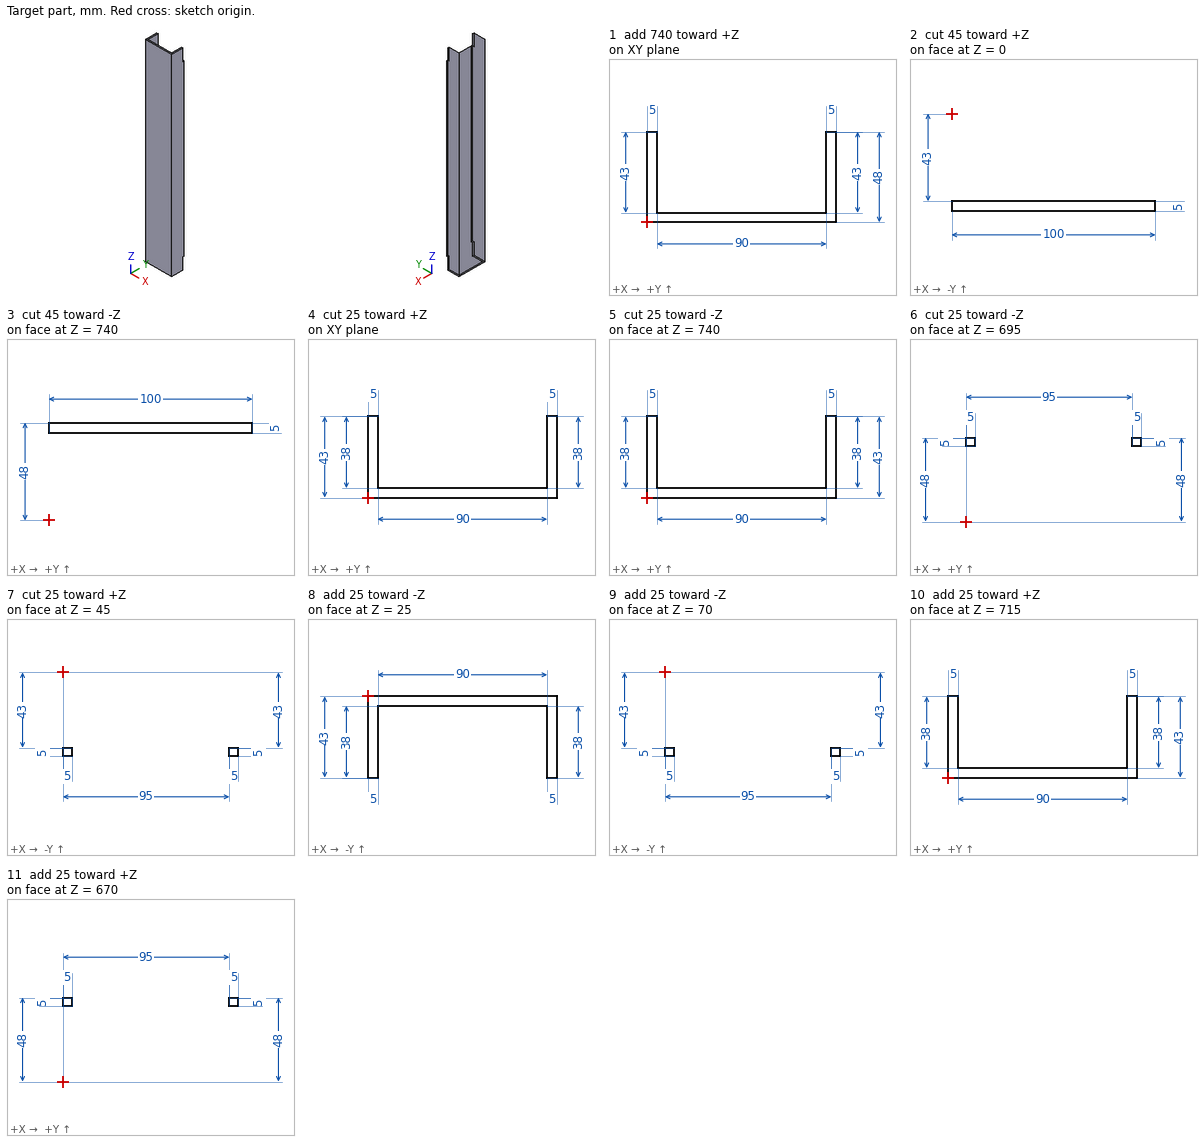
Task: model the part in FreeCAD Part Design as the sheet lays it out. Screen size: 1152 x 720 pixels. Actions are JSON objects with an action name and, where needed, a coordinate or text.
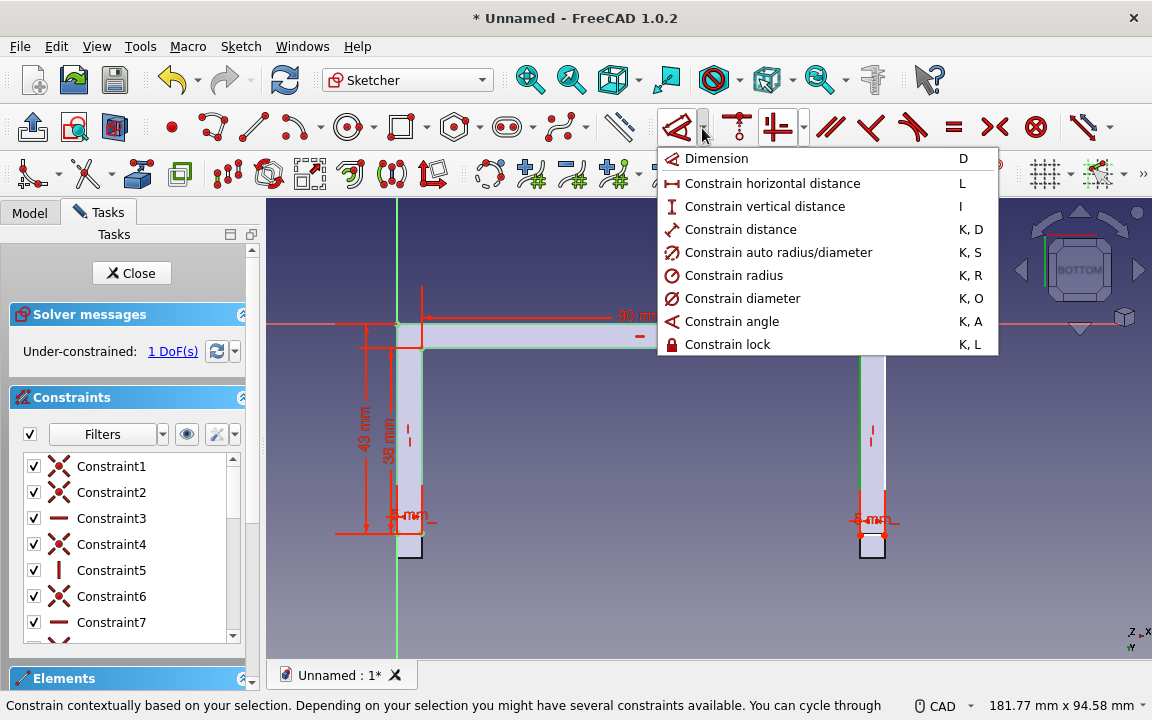
{"action": "left_click", "coordinate": [828, 206]}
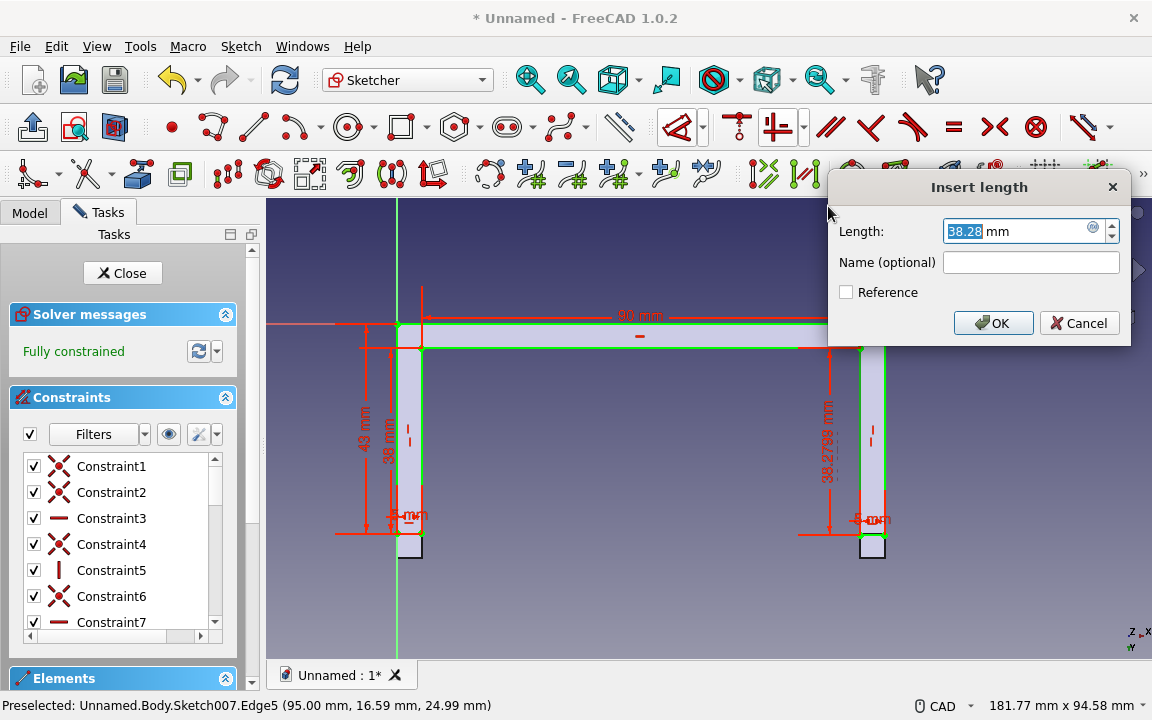
{"action": "type", "text": "38"}
{"action": "key", "text": "Return"}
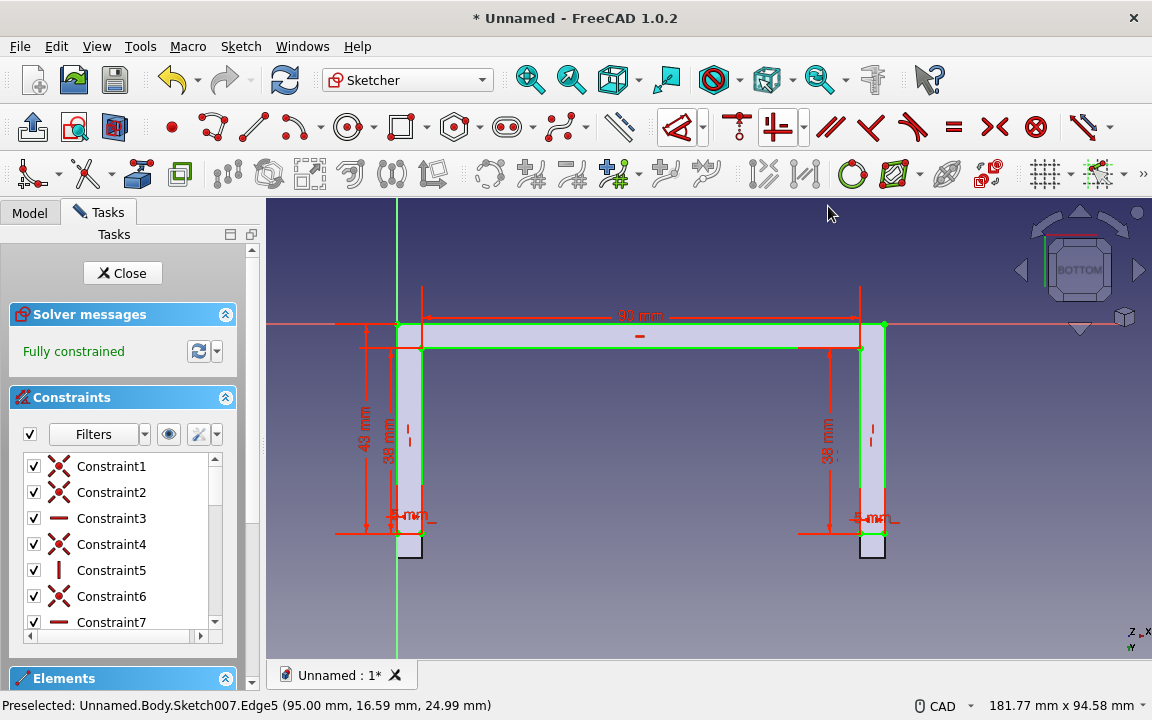
{"action": "left_click", "coordinate": [123, 273]}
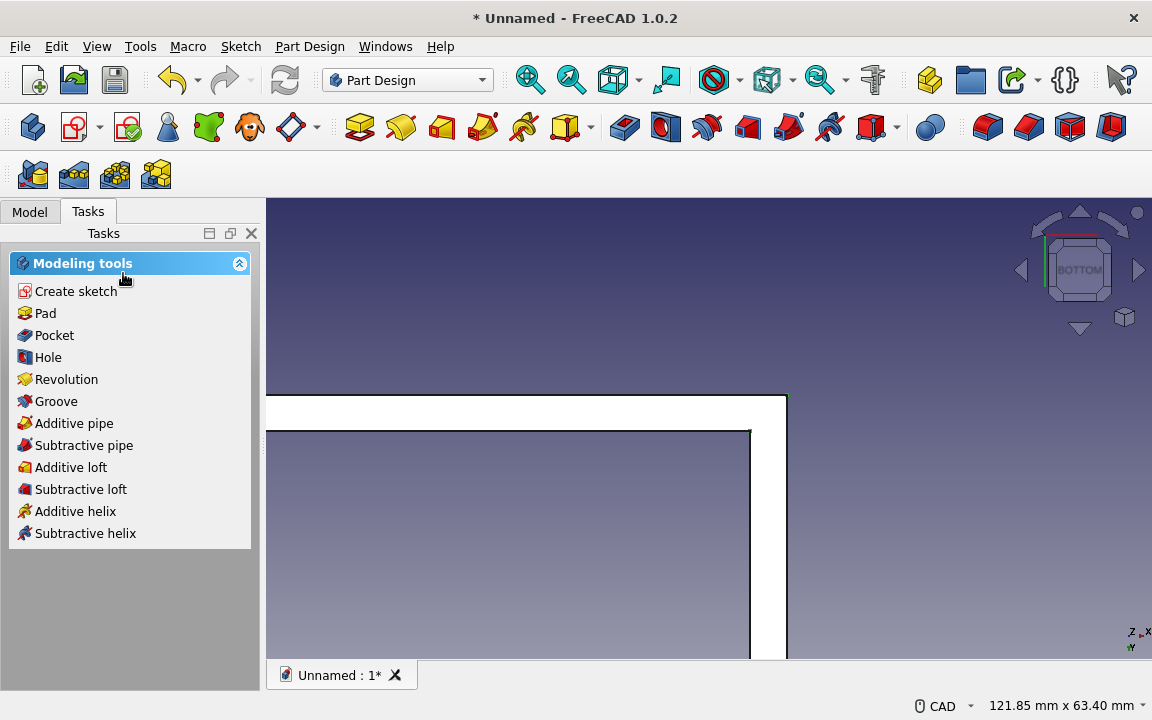
{"action": "left_click", "coordinate": [360, 128]}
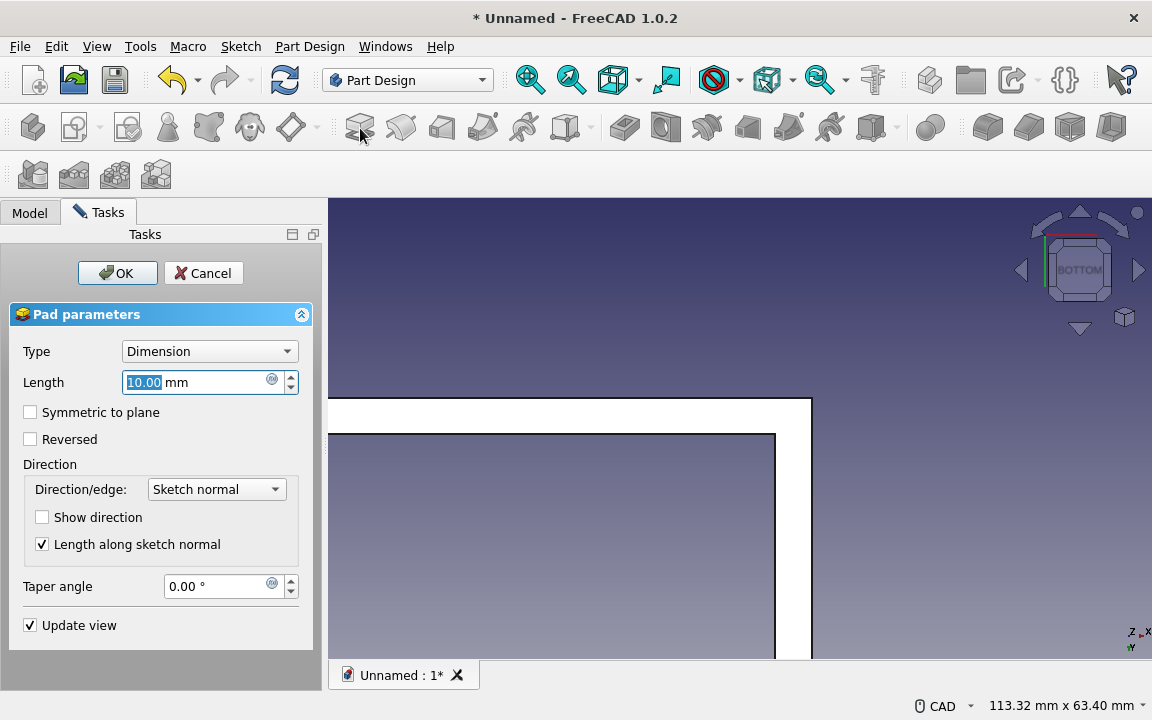
{"action": "type", "text": "25"}
{"action": "key", "text": "Tab"}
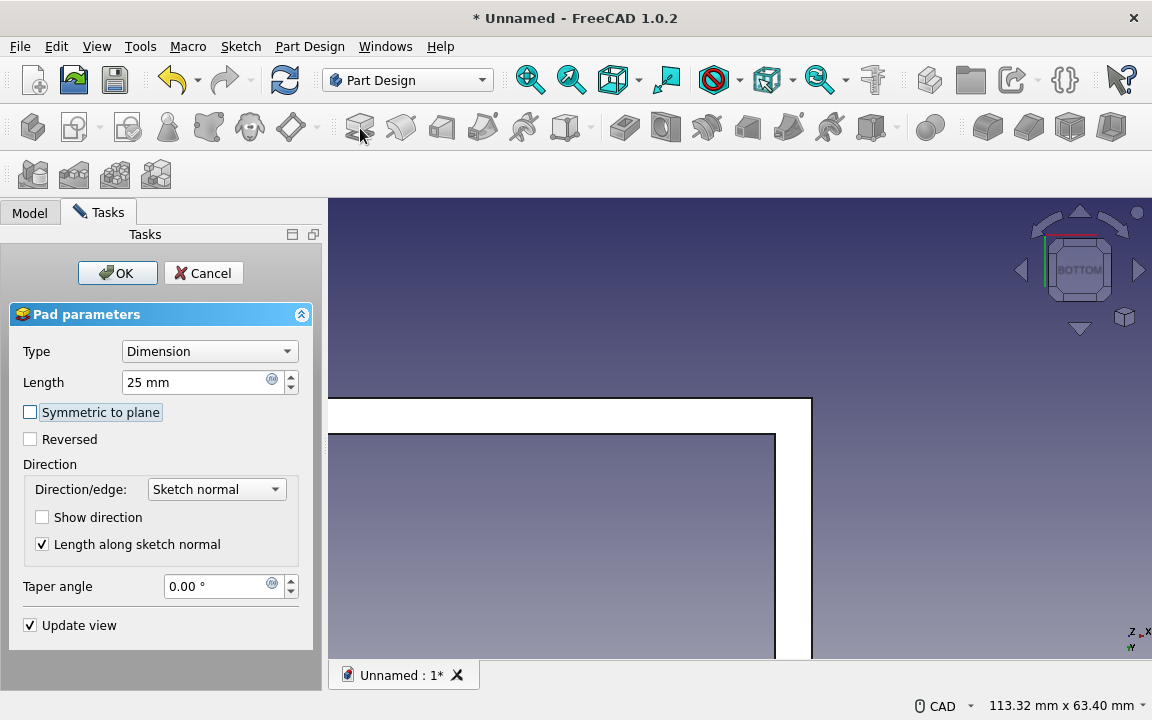
{"action": "left_click", "coordinate": [118, 273]}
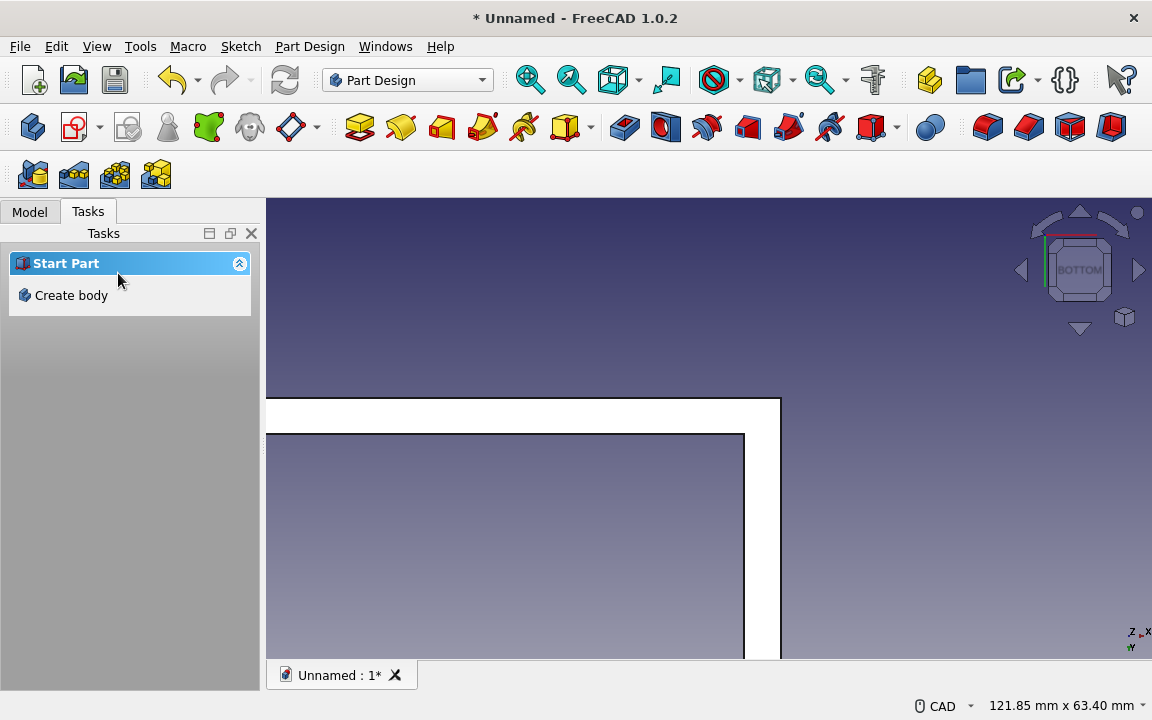
{"action": "left_click", "coordinate": [531, 80]}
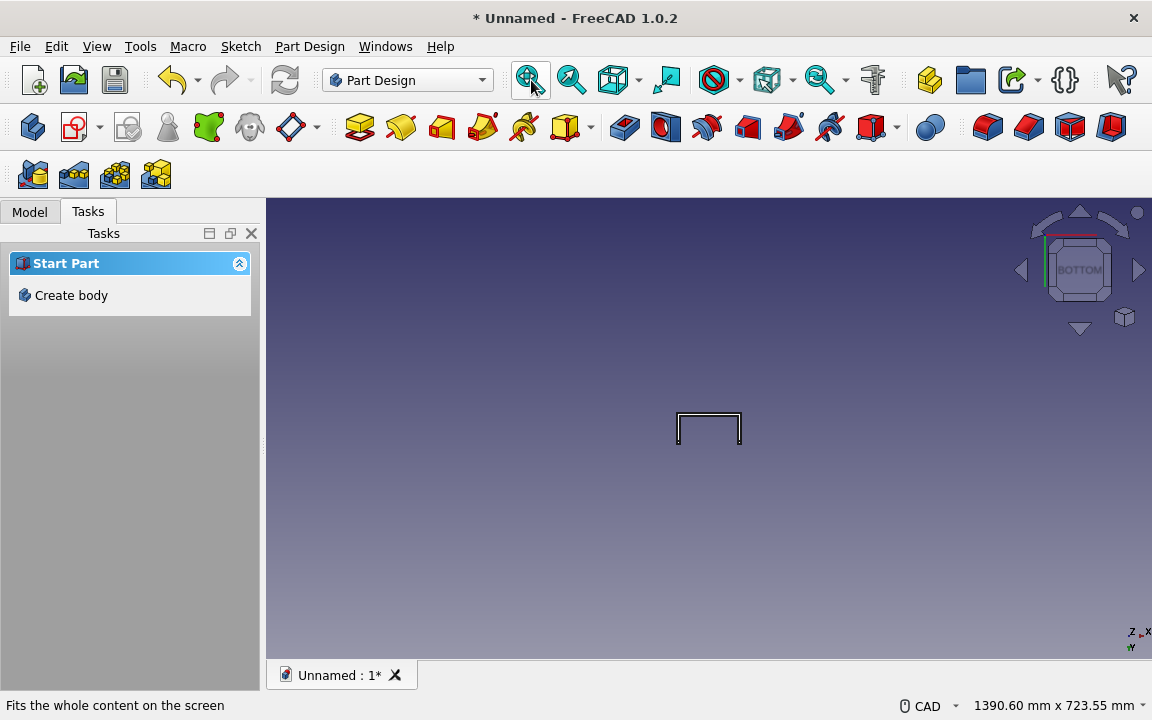
{"action": "scroll", "coordinate": [679, 441], "scroll_direction": "up", "scroll_amount": 11}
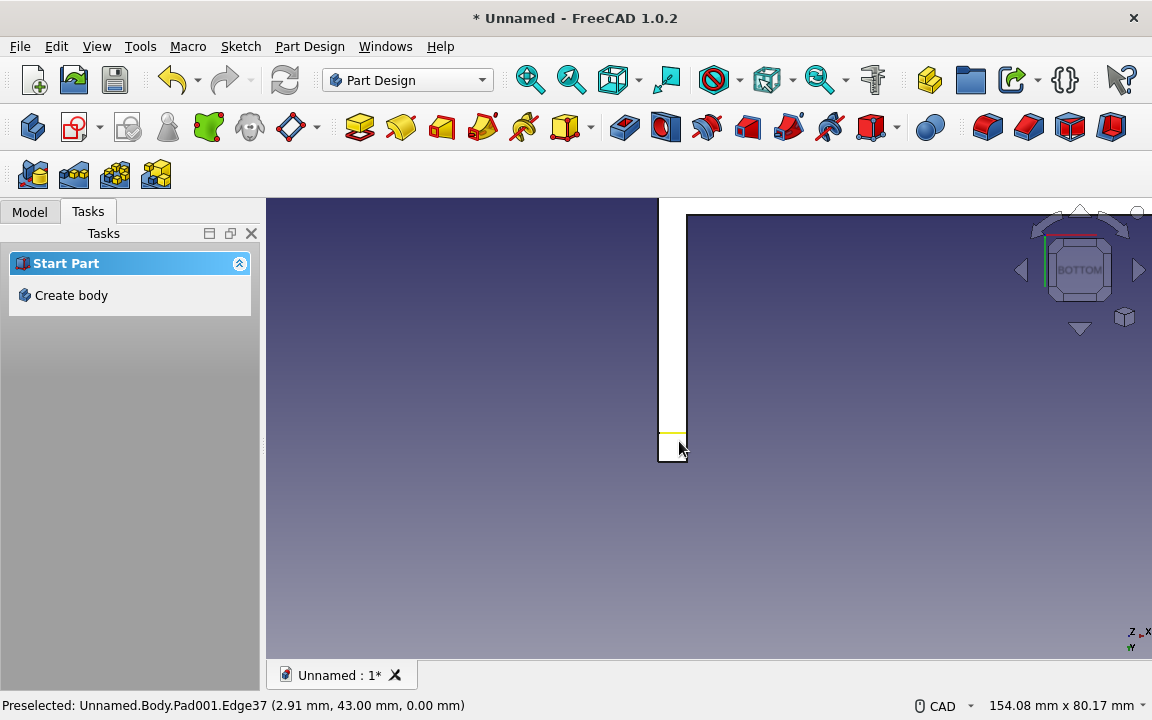
{"action": "left_click", "coordinate": [673, 447]}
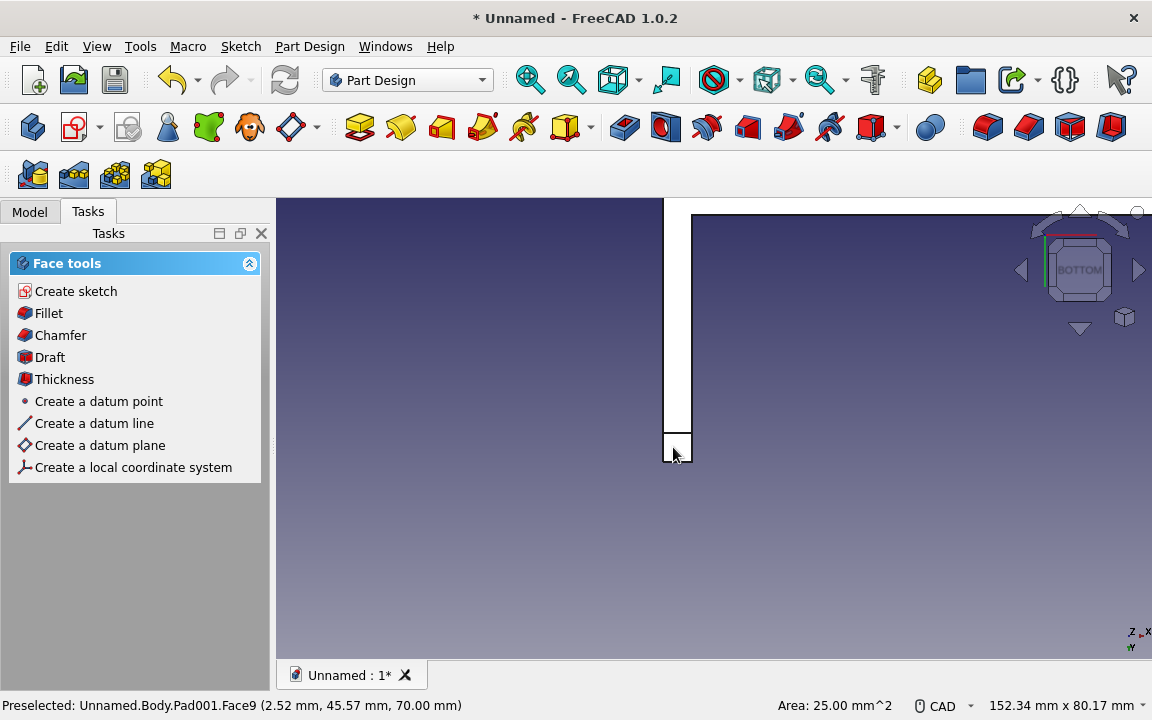
{"action": "left_click", "coordinate": [74, 128]}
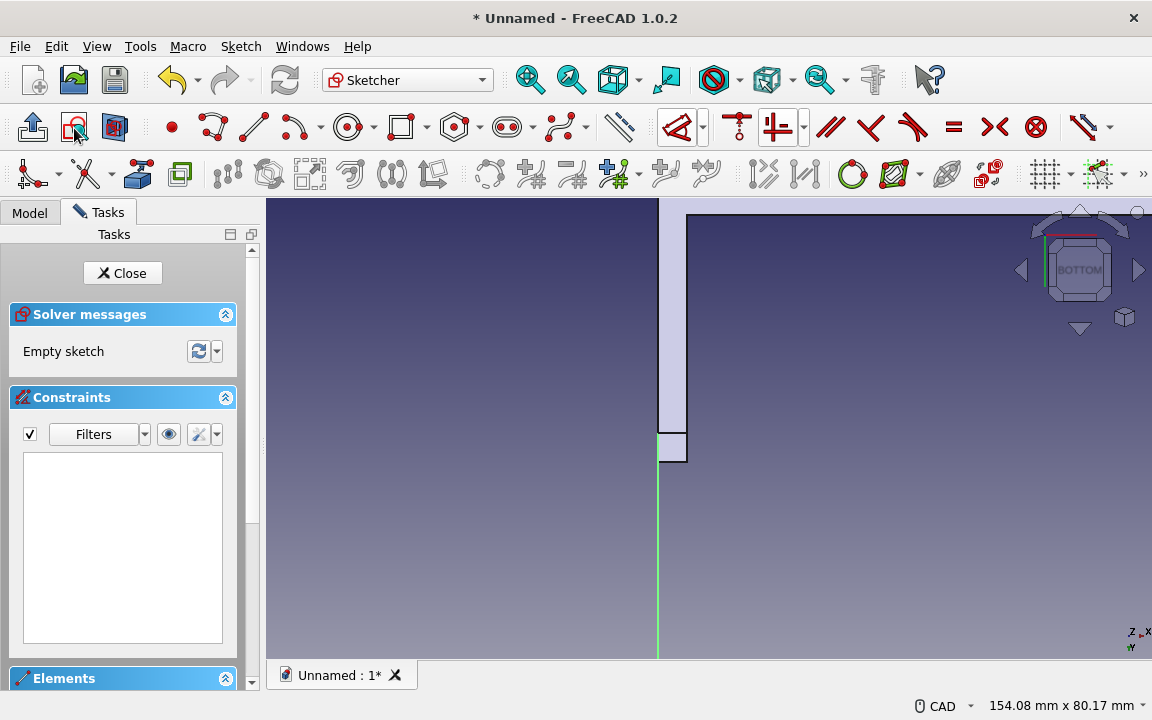
{"action": "left_click", "coordinate": [115, 128]}